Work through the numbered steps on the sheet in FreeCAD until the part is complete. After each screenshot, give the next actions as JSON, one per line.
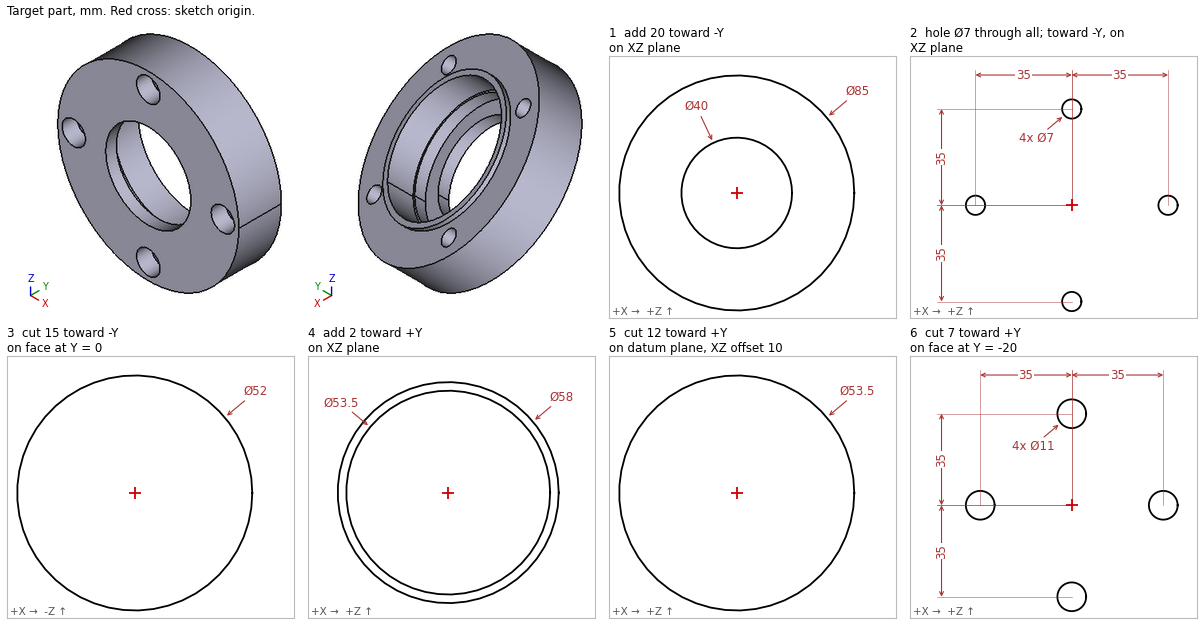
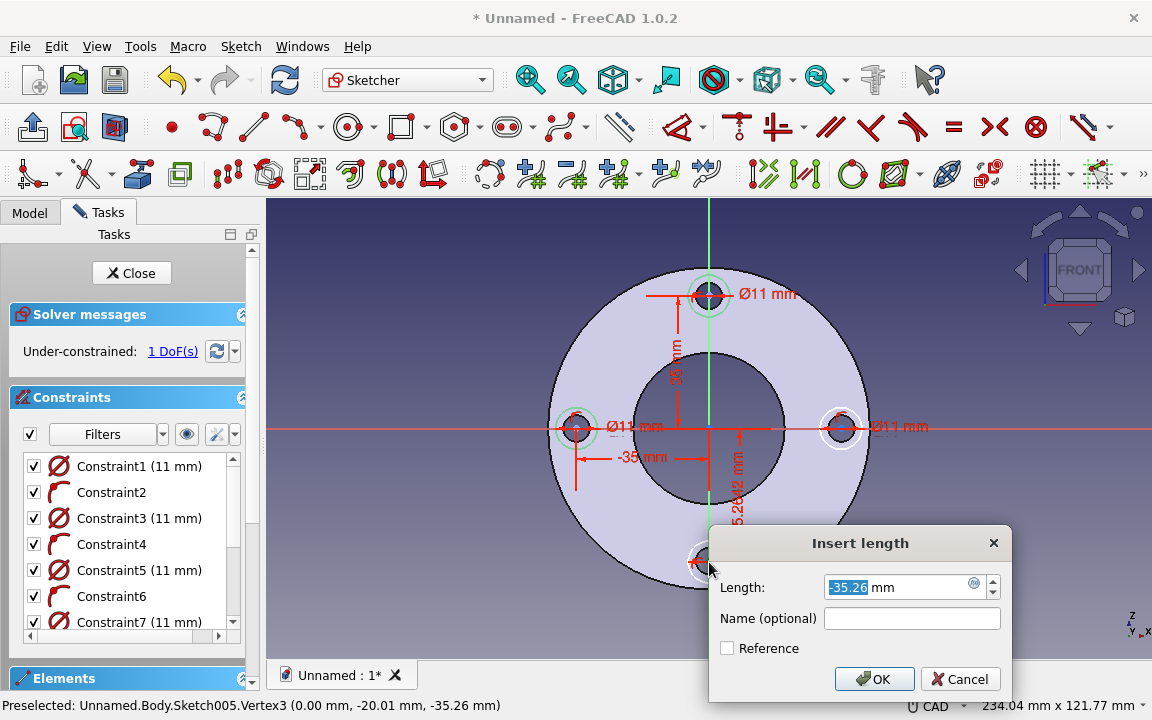
{"action": "type", "text": "-35"}
{"action": "key", "text": "Return"}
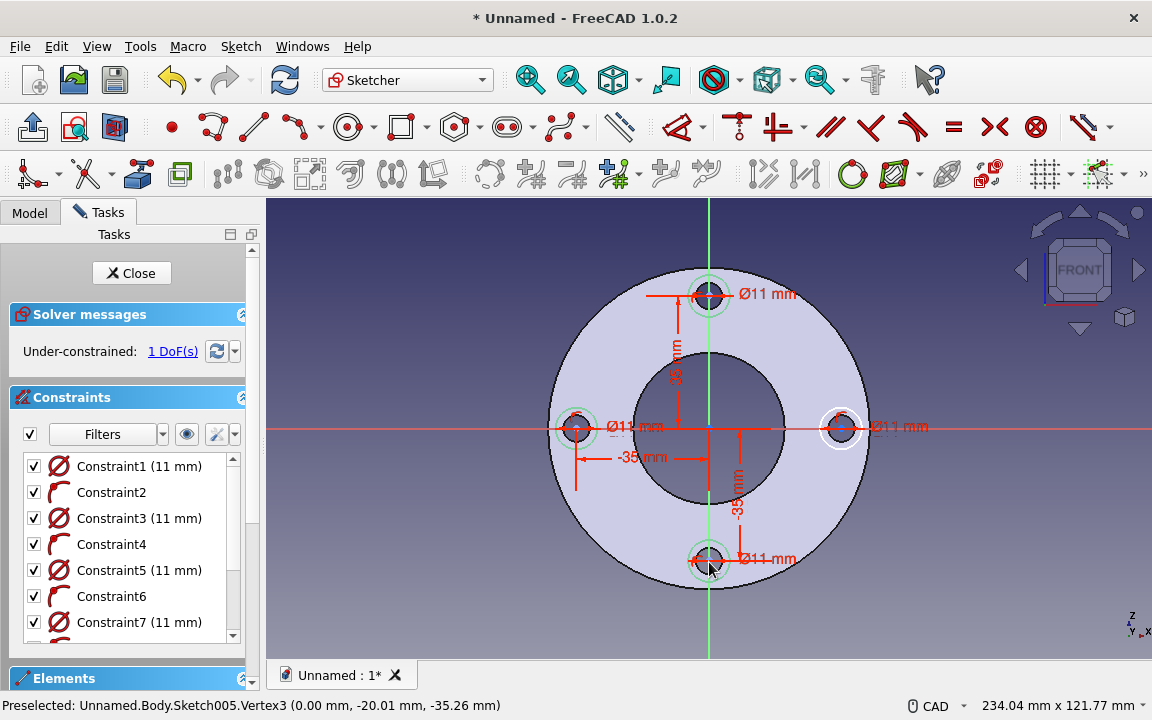
{"action": "left_click", "coordinate": [841, 428]}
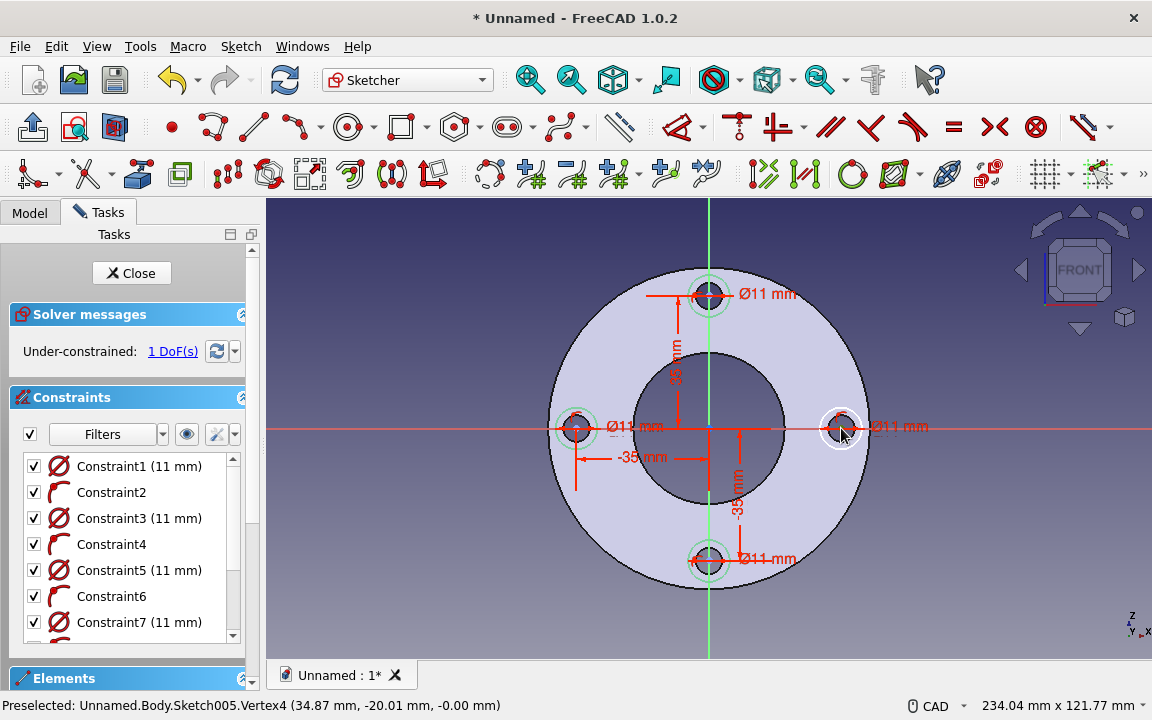
{"action": "left_click", "coordinate": [702, 128]}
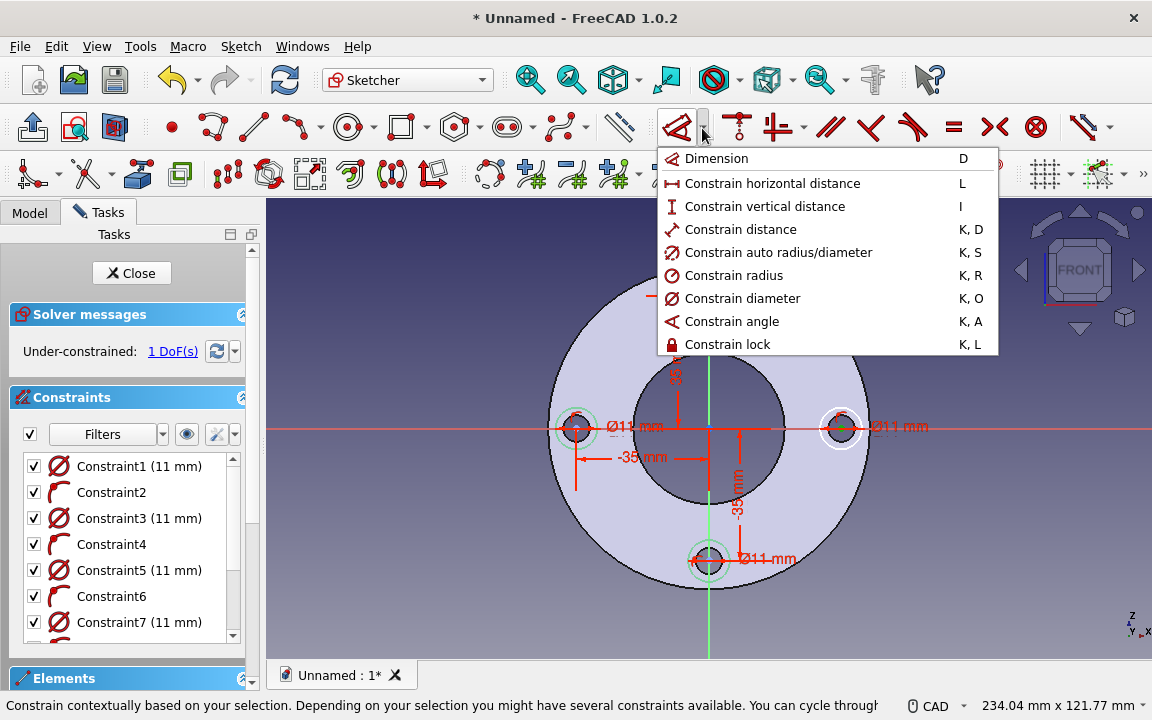
{"action": "left_click", "coordinate": [828, 184]}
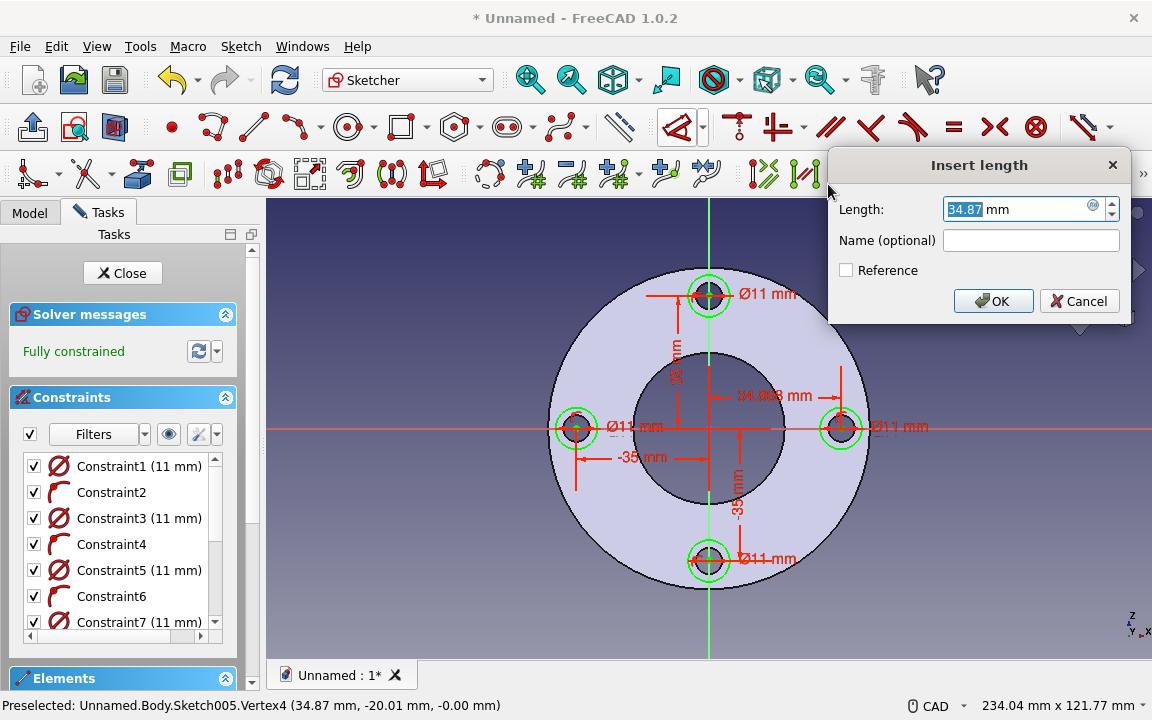
{"action": "type", "text": "35"}
{"action": "key", "text": "Return"}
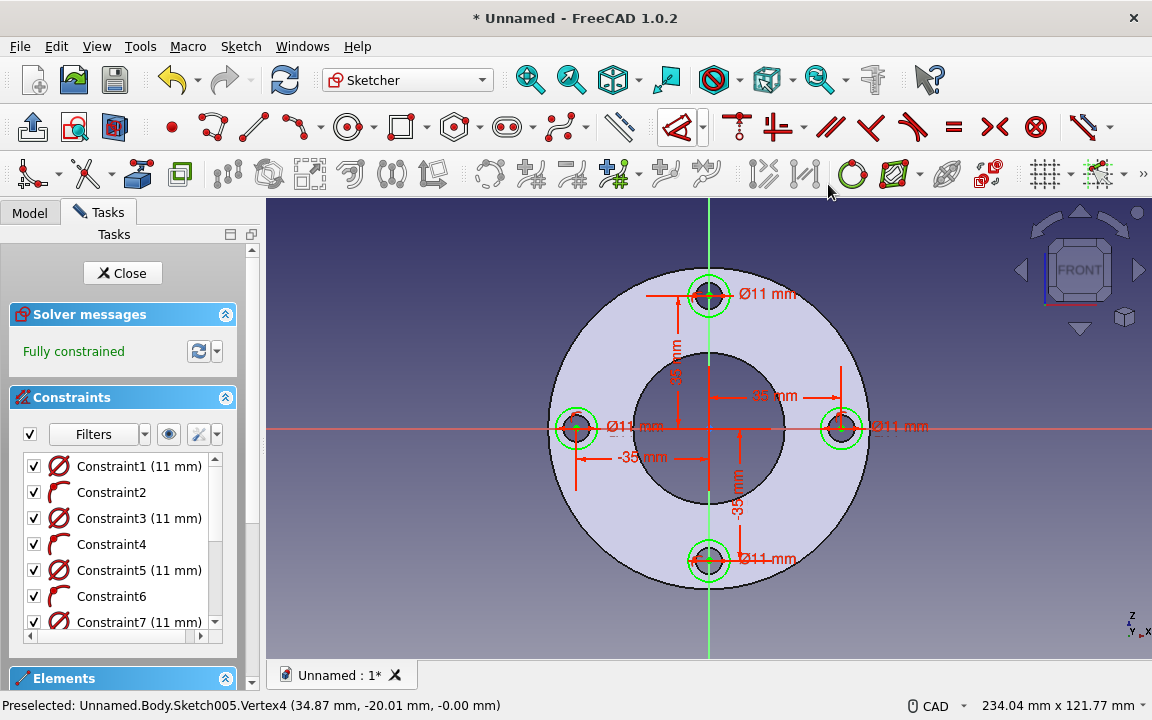
{"action": "left_click", "coordinate": [123, 273]}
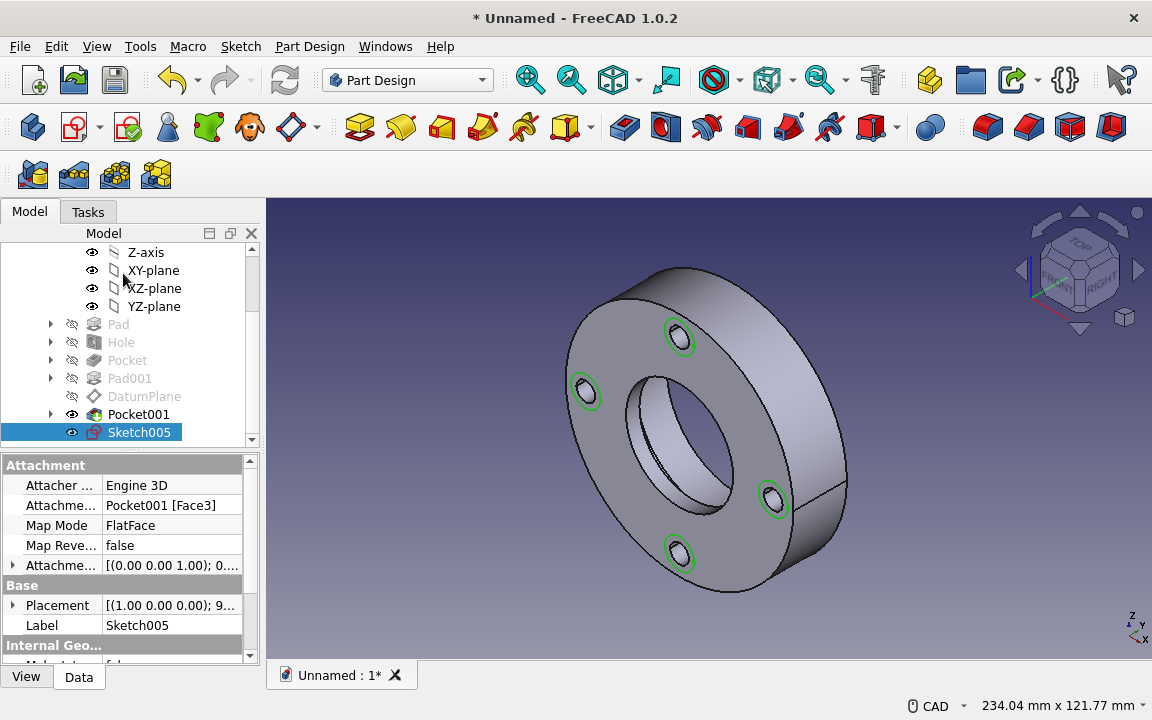
{"action": "left_click", "coordinate": [625, 128]}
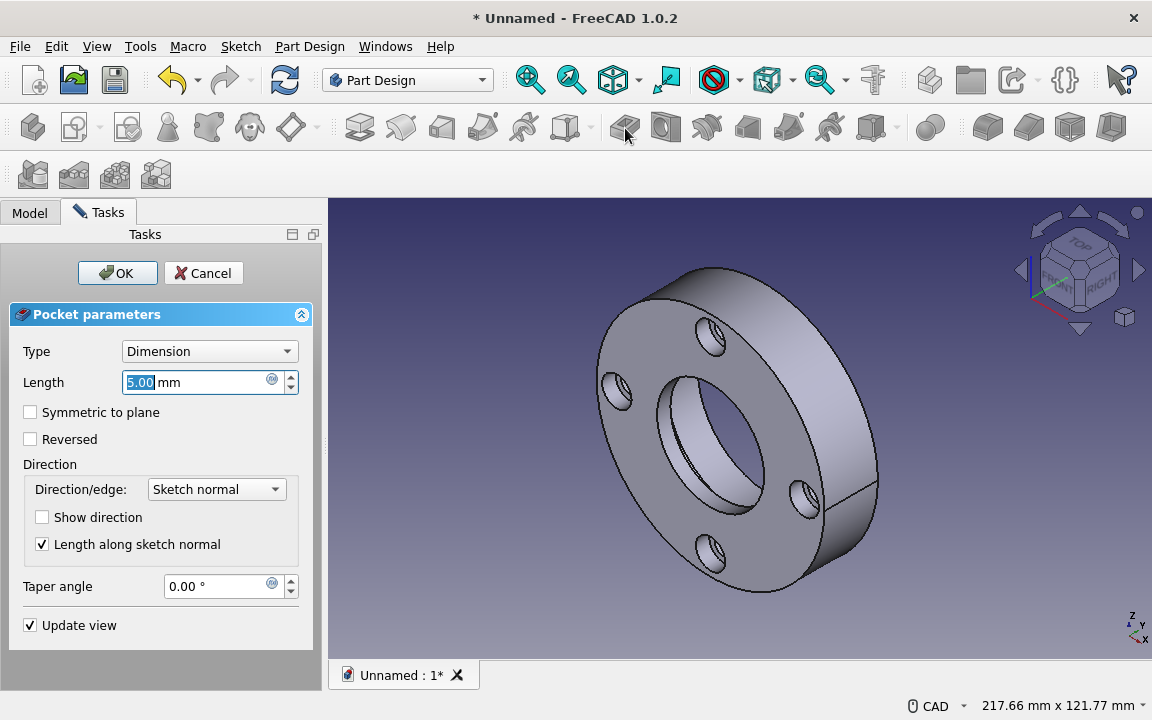
{"action": "type", "text": "7"}
{"action": "key", "text": "Tab"}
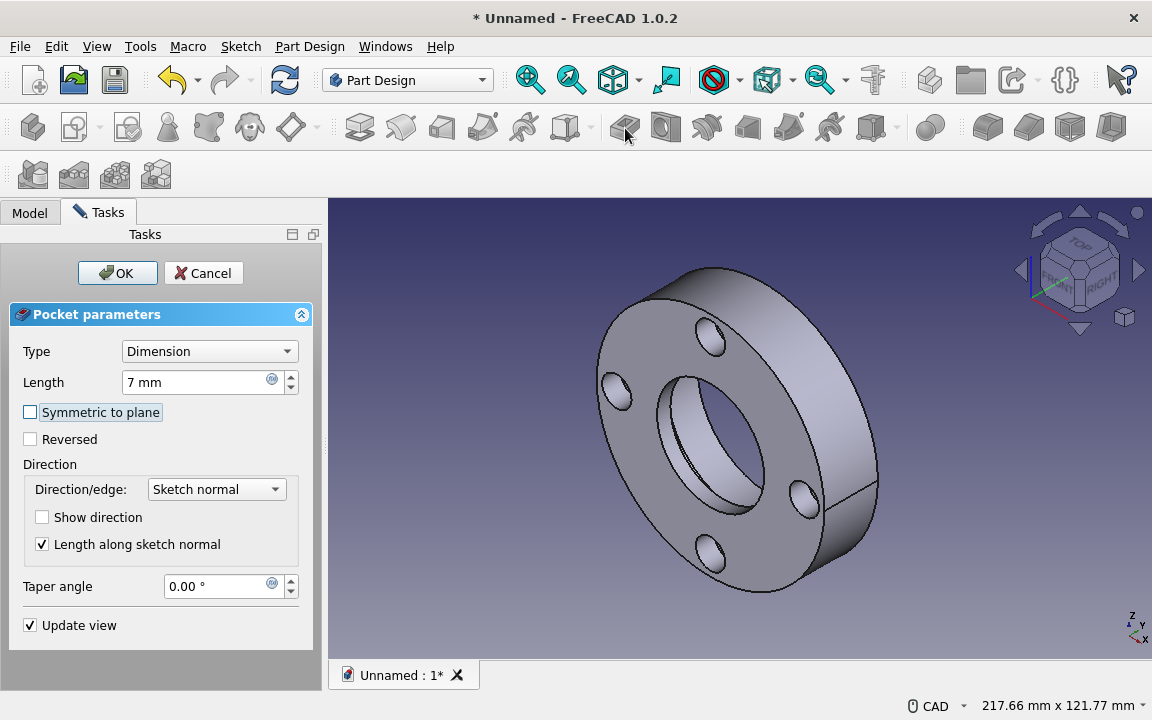
{"action": "left_click", "coordinate": [118, 273]}